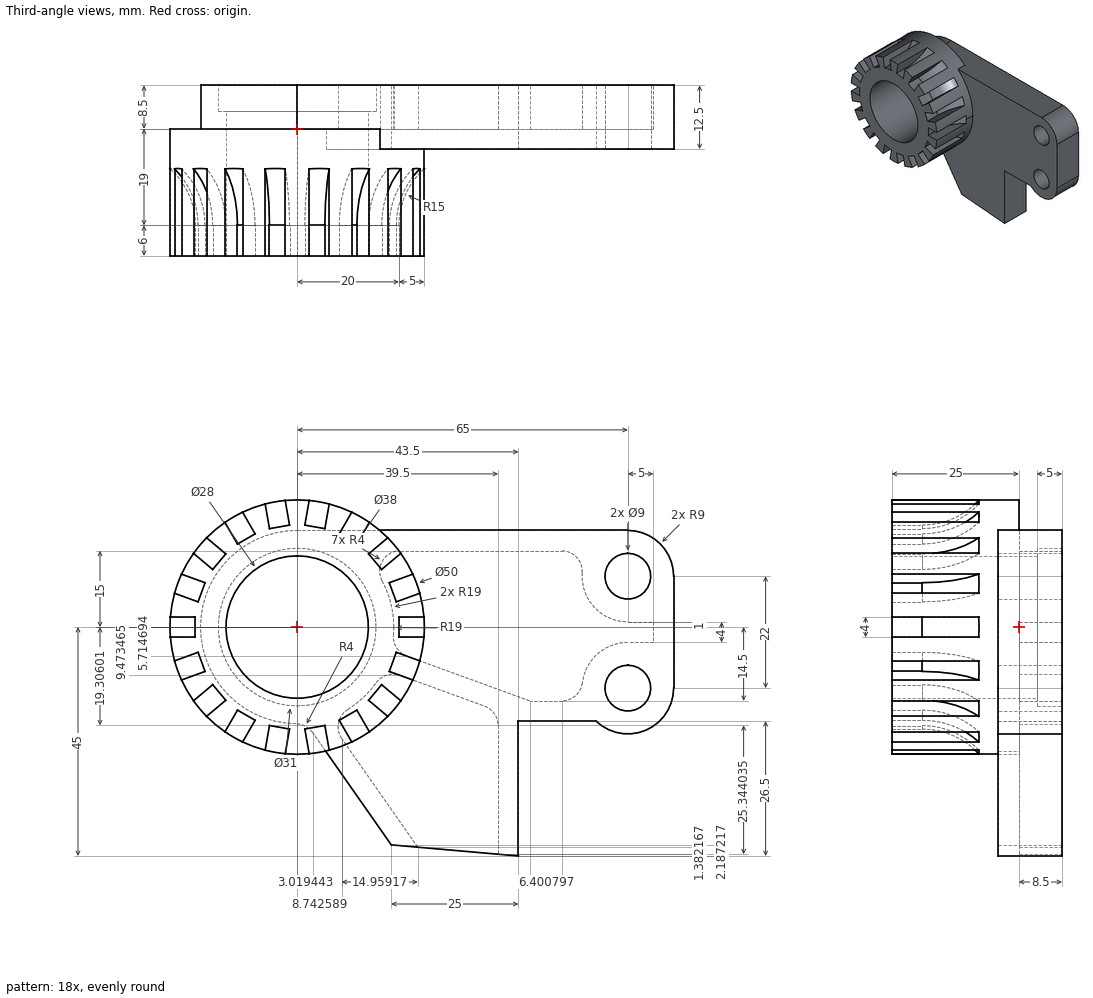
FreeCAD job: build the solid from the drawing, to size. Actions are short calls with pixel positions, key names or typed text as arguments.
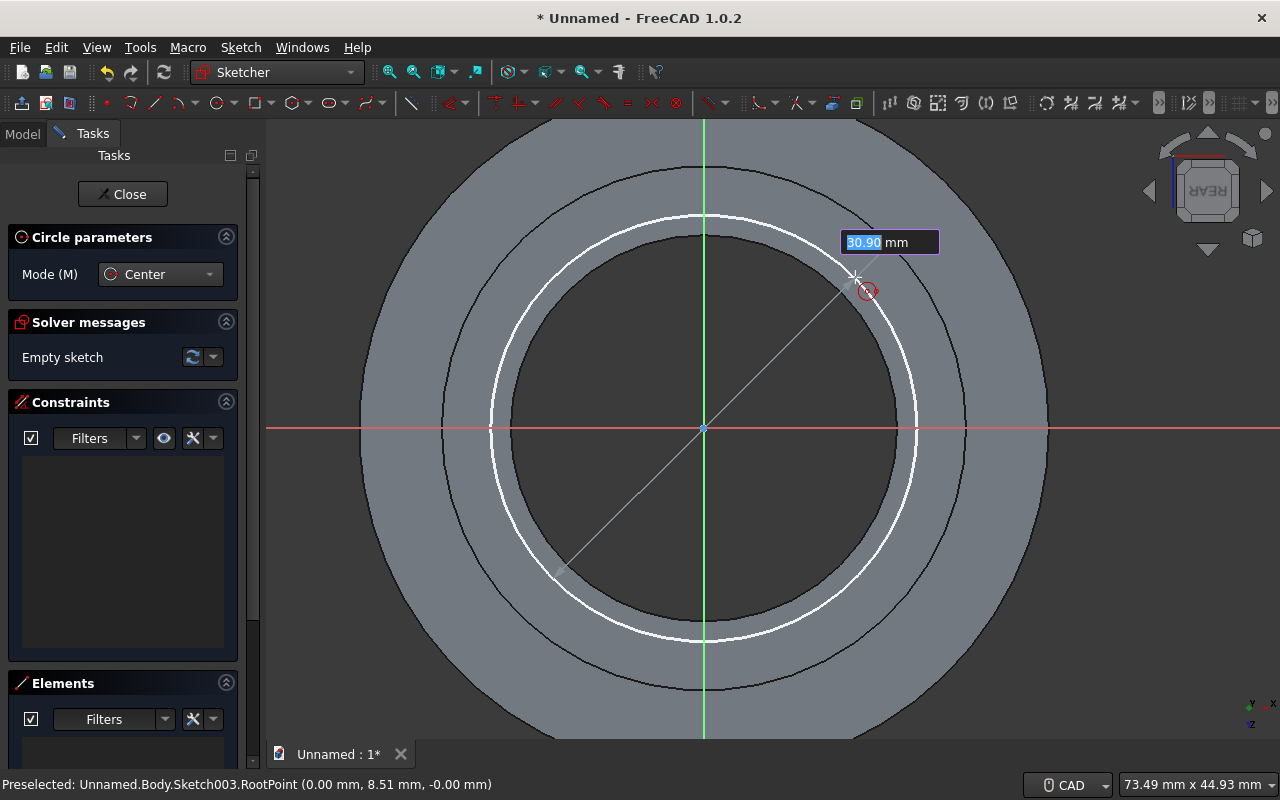
text(31)
key(Return)
key(Escape)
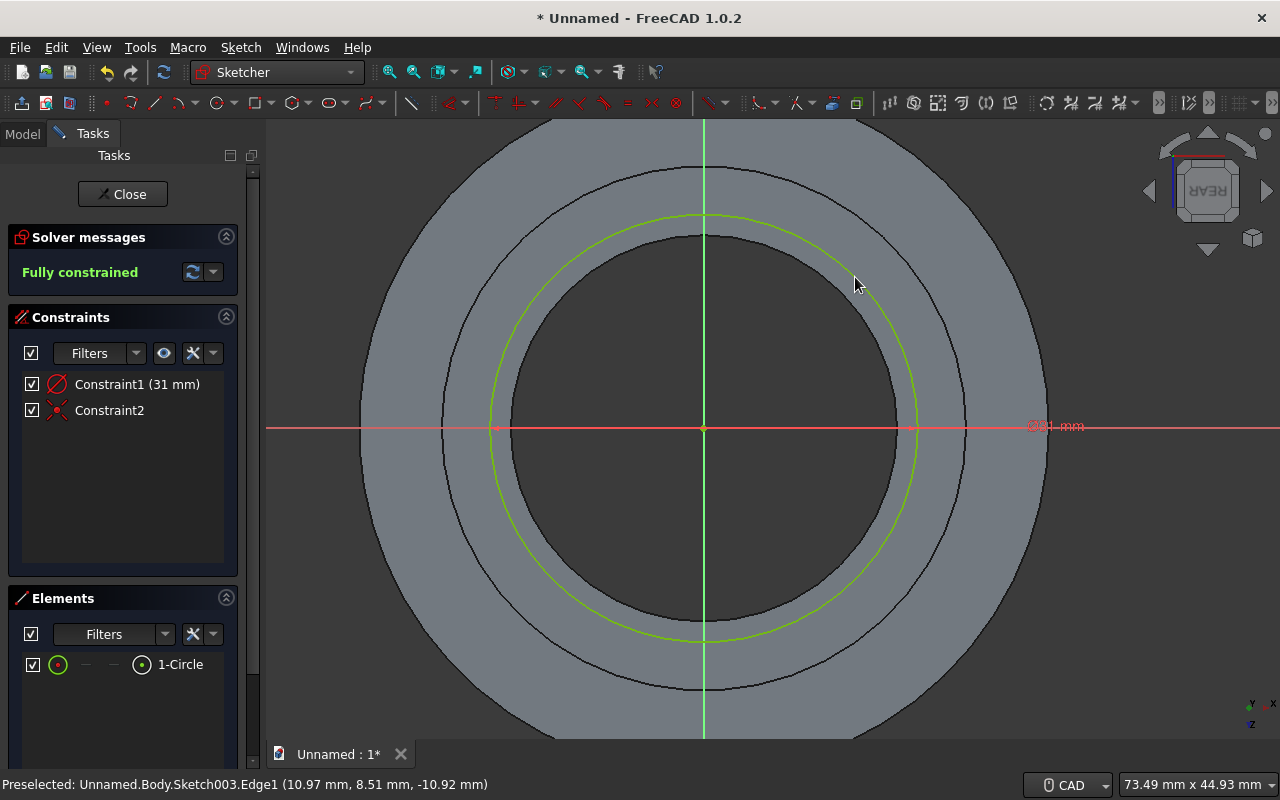
click(123, 194)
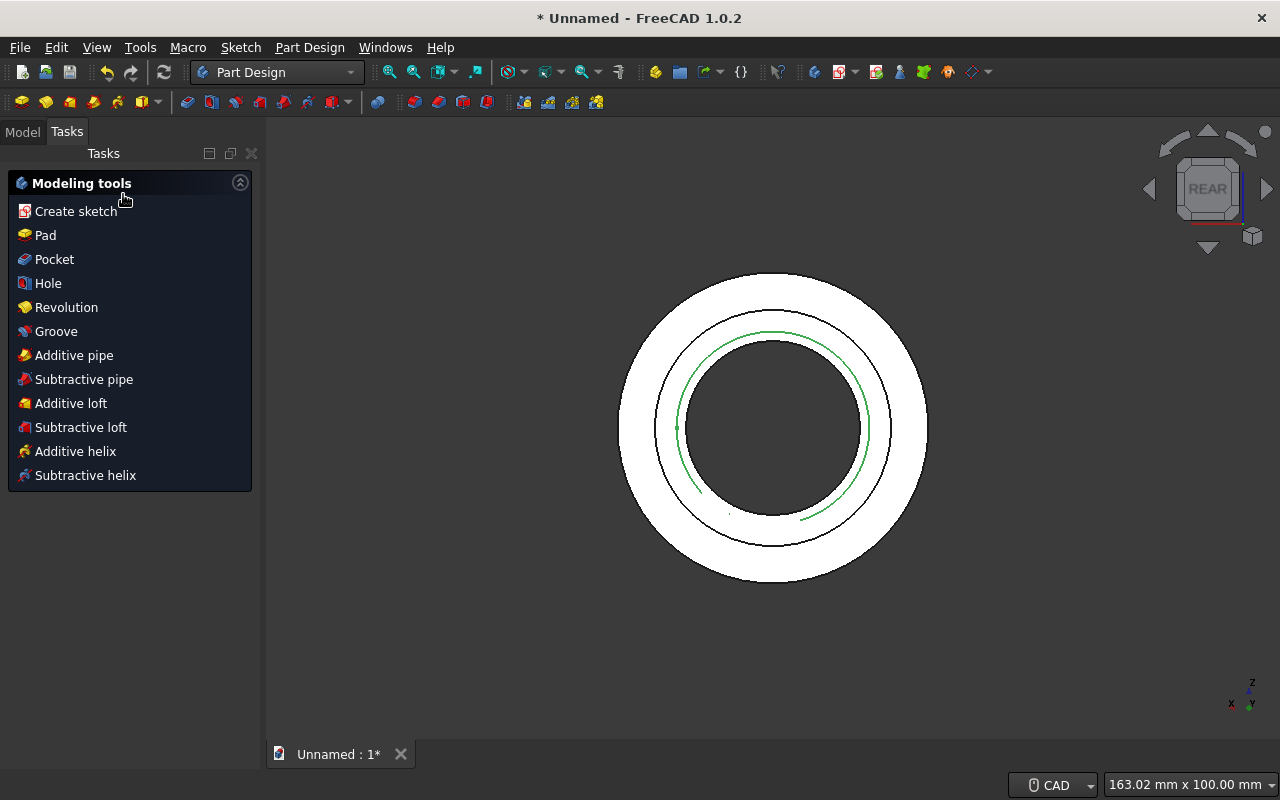
click(188, 102)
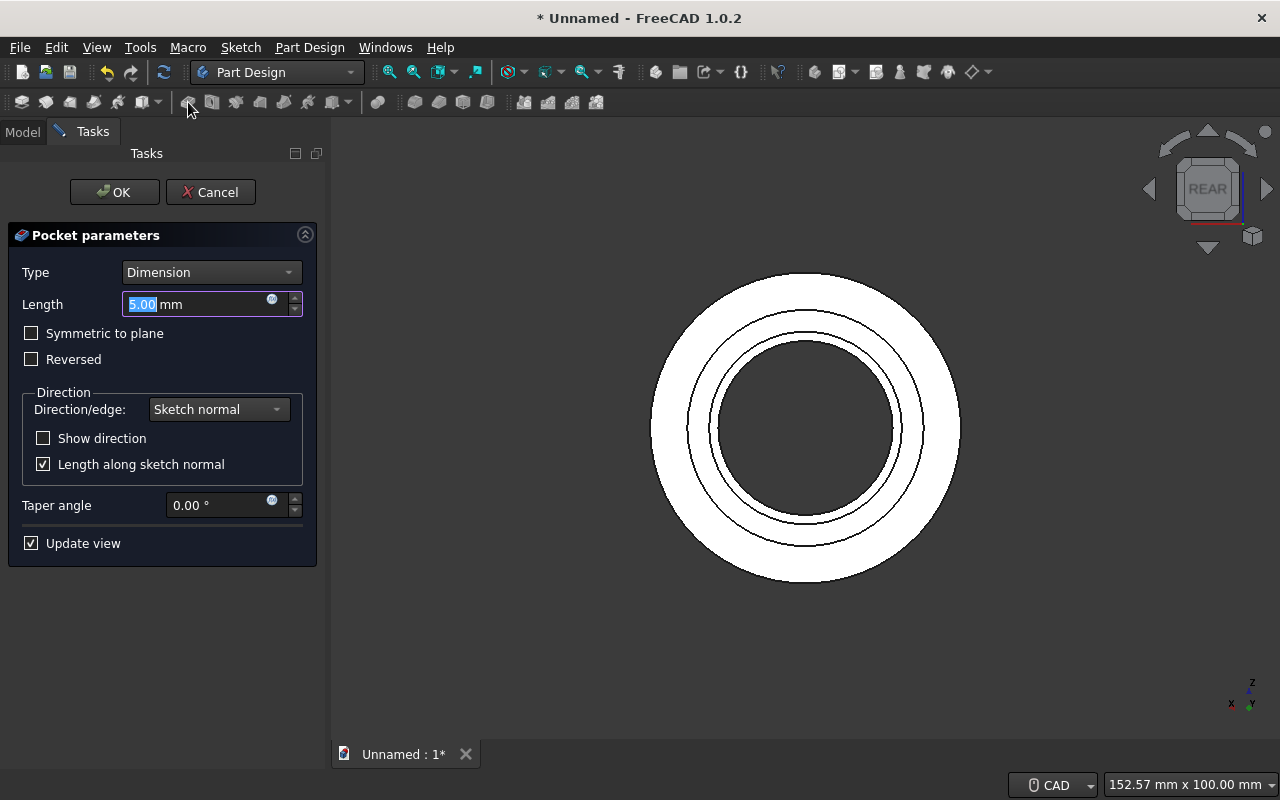
text(5)
key(Tab)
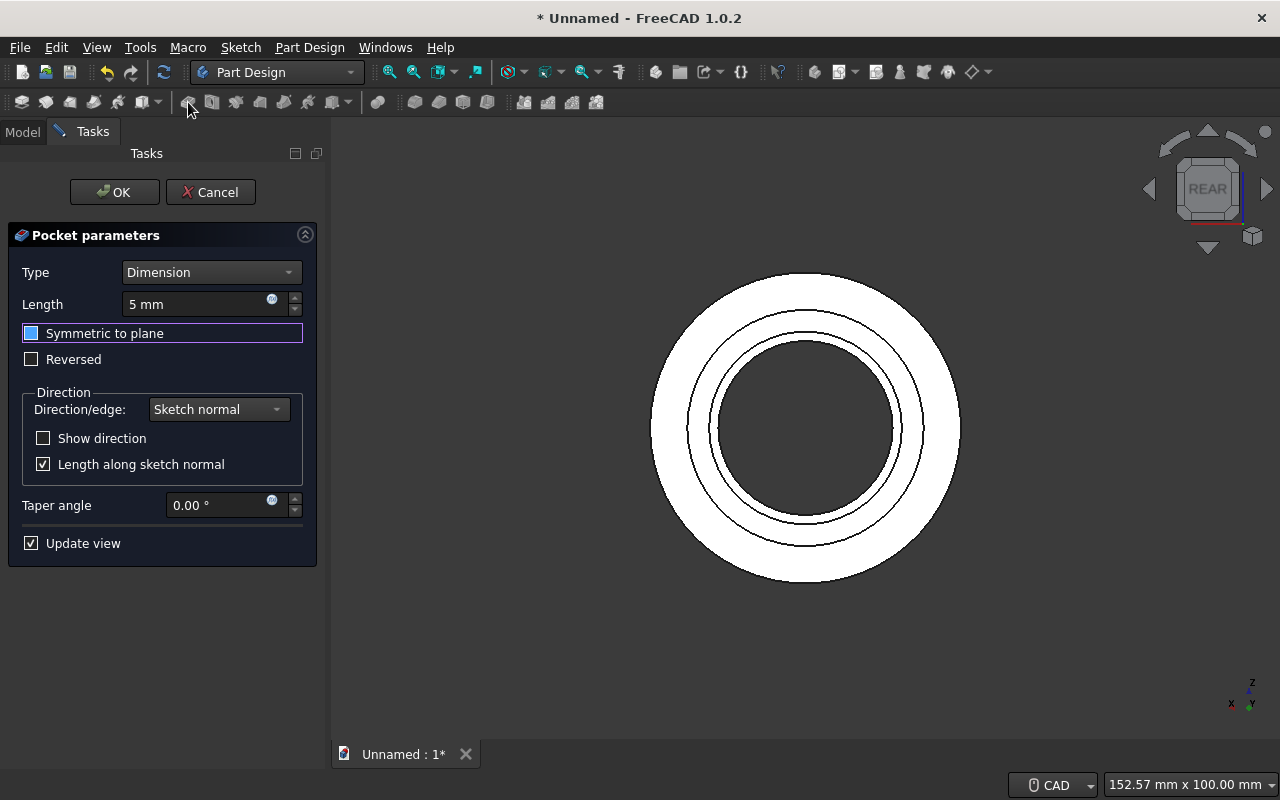
click(115, 192)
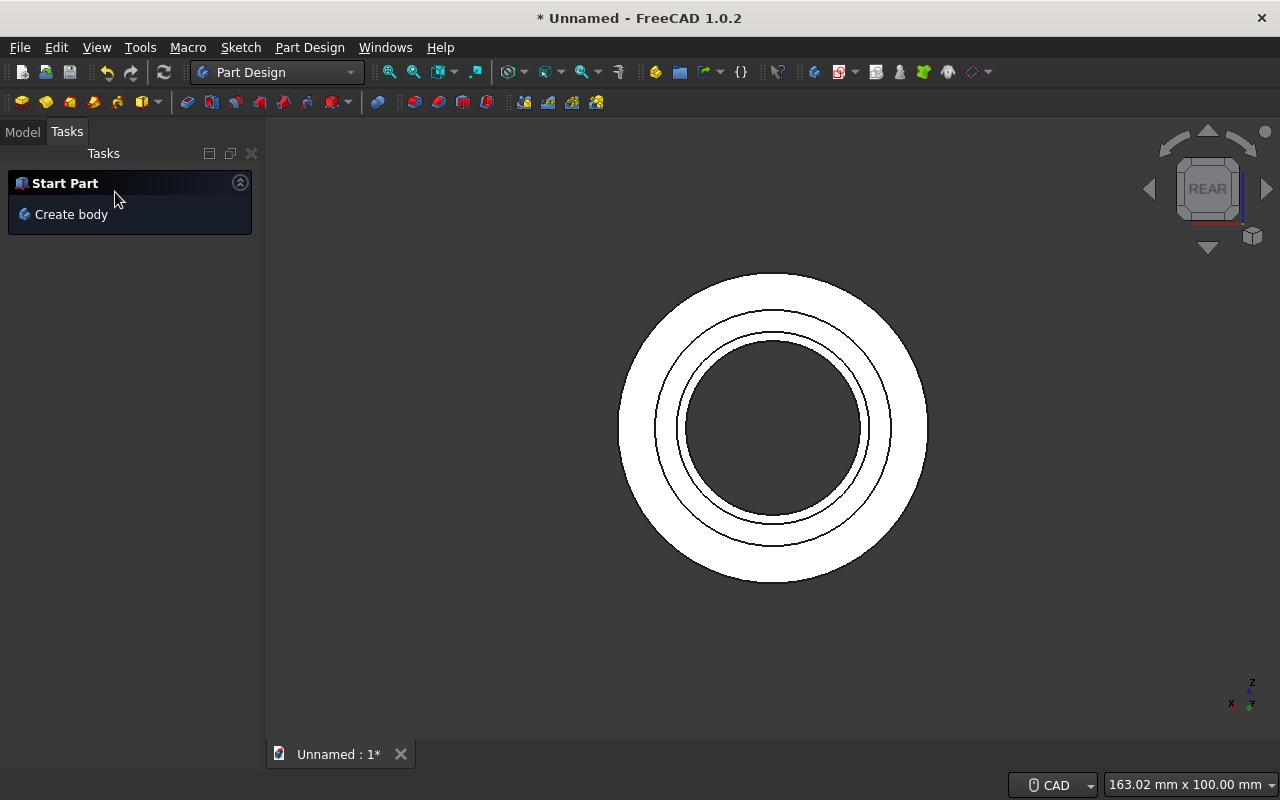
click(23, 131)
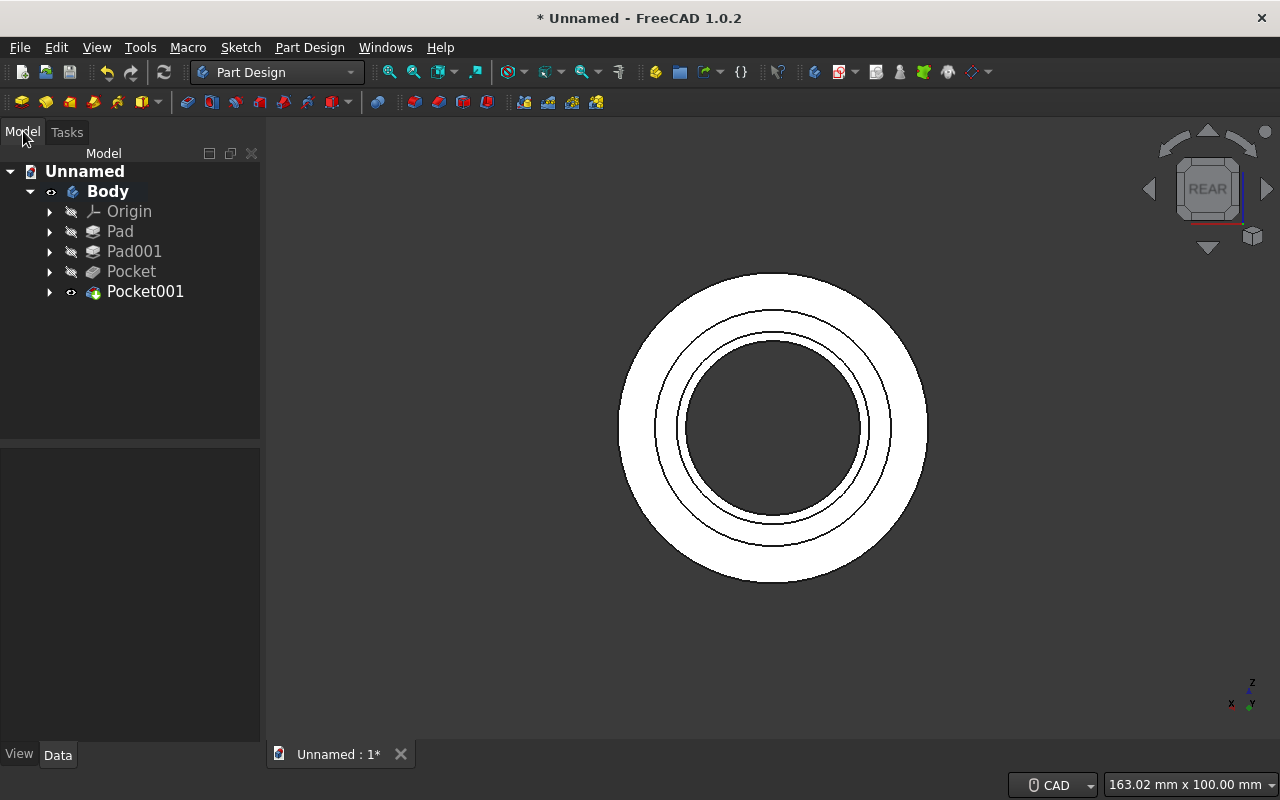
click(50, 212)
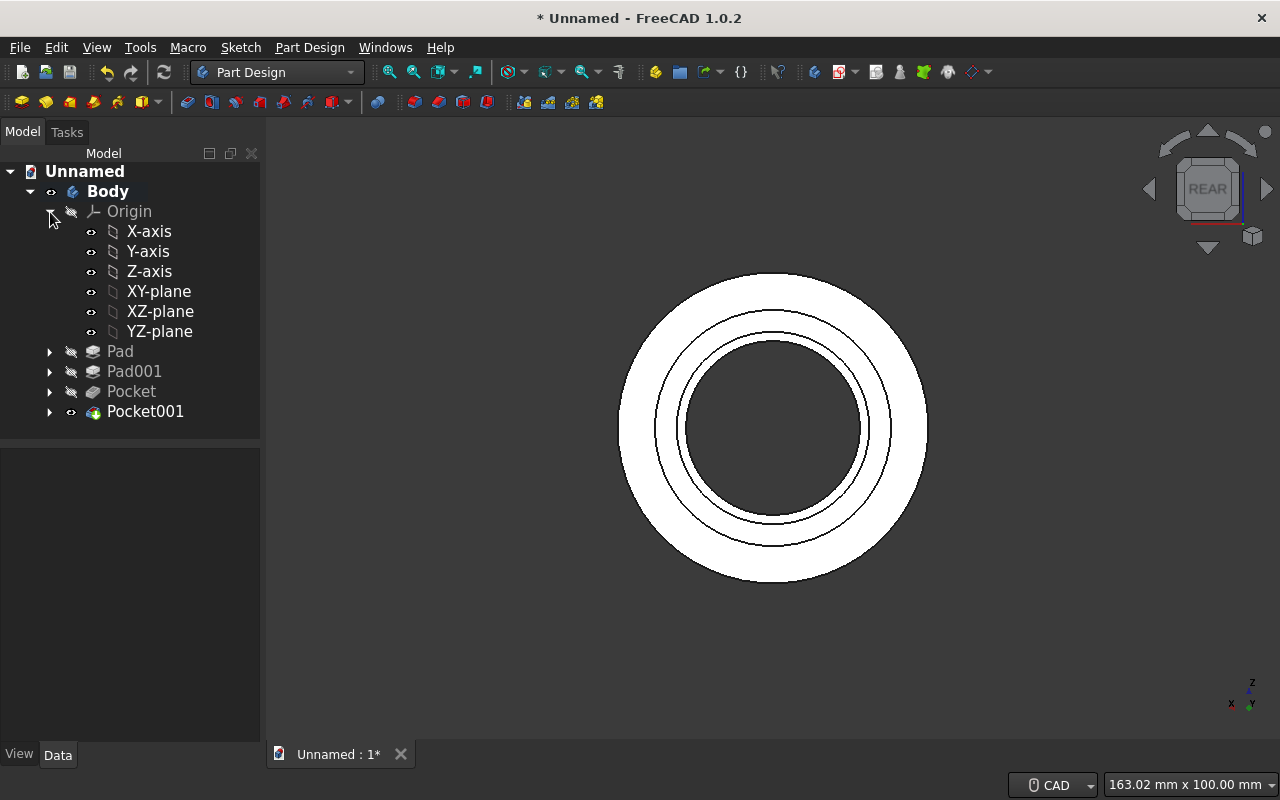
click(136, 312)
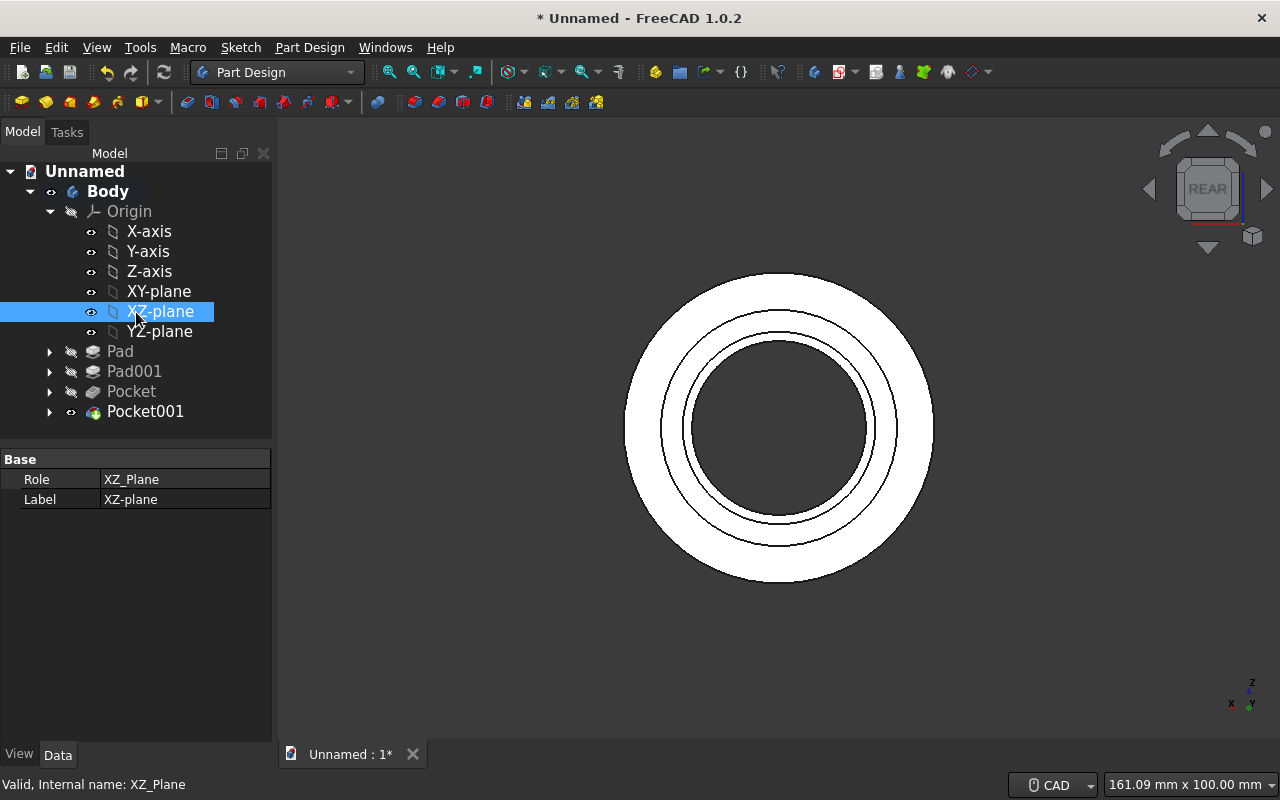
click(972, 72)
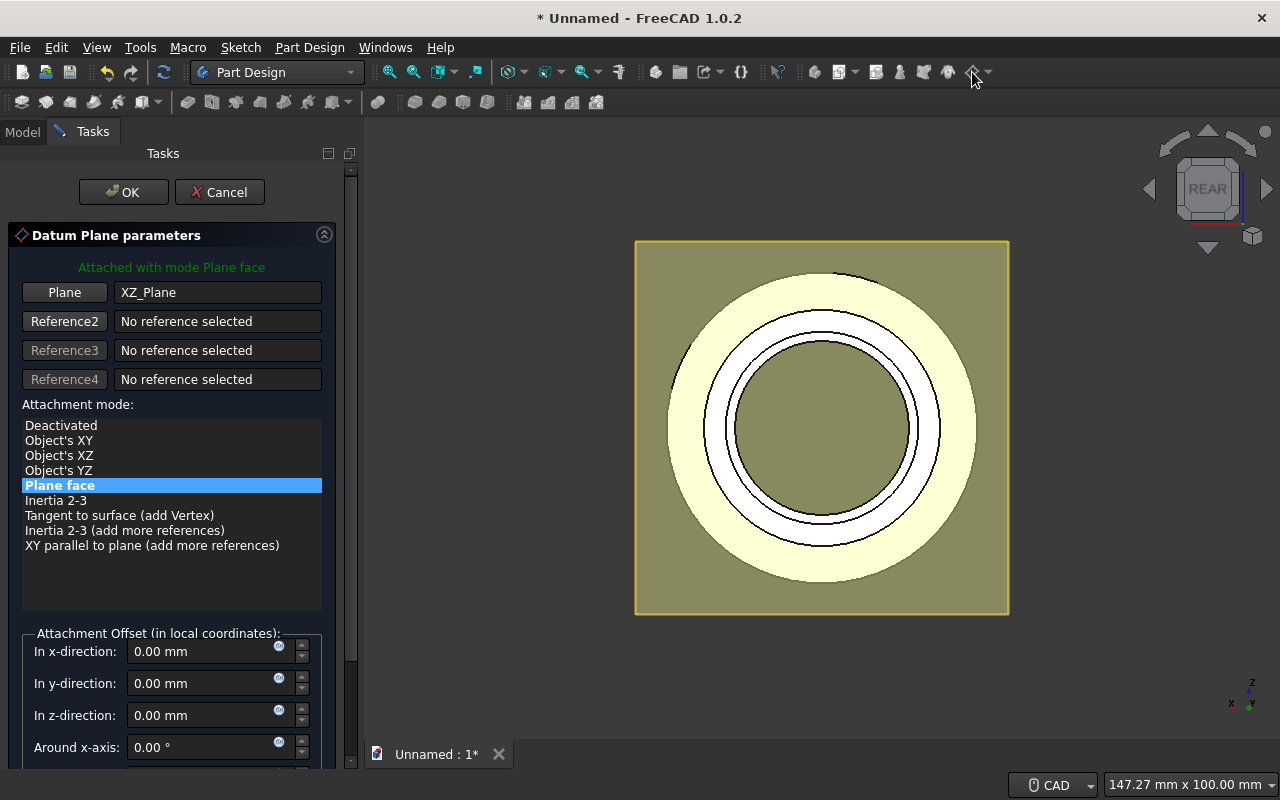
triple_click(210, 715)